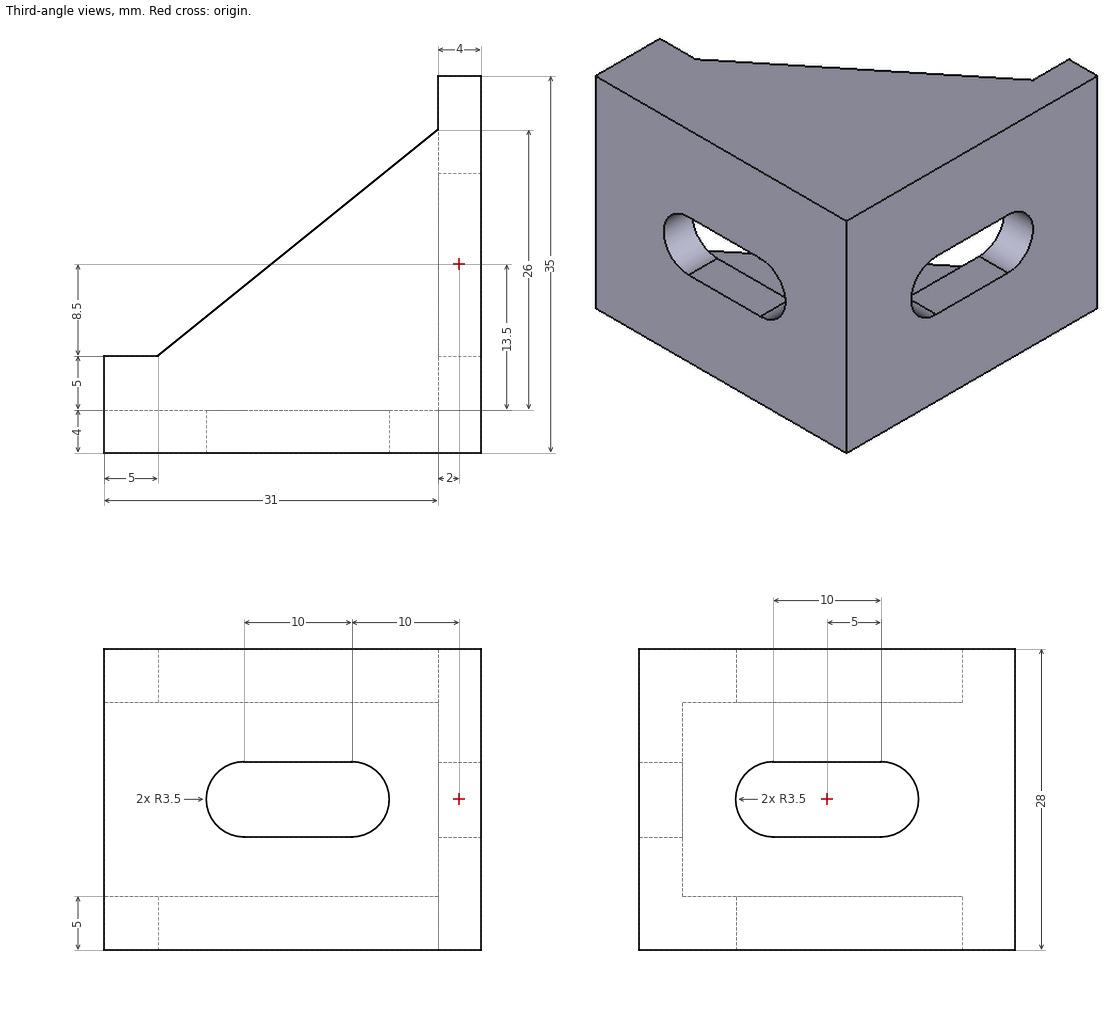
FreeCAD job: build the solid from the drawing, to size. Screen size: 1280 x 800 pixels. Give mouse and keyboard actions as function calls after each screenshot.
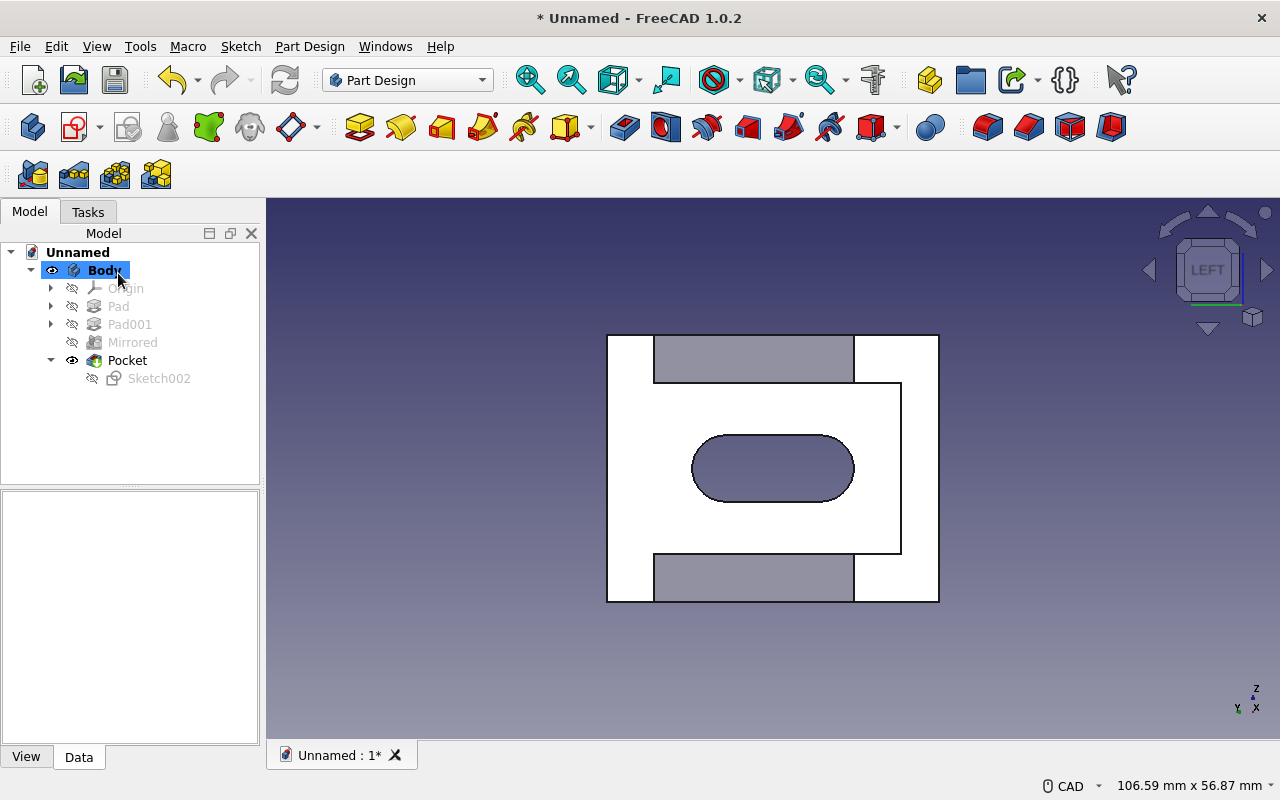
key(4)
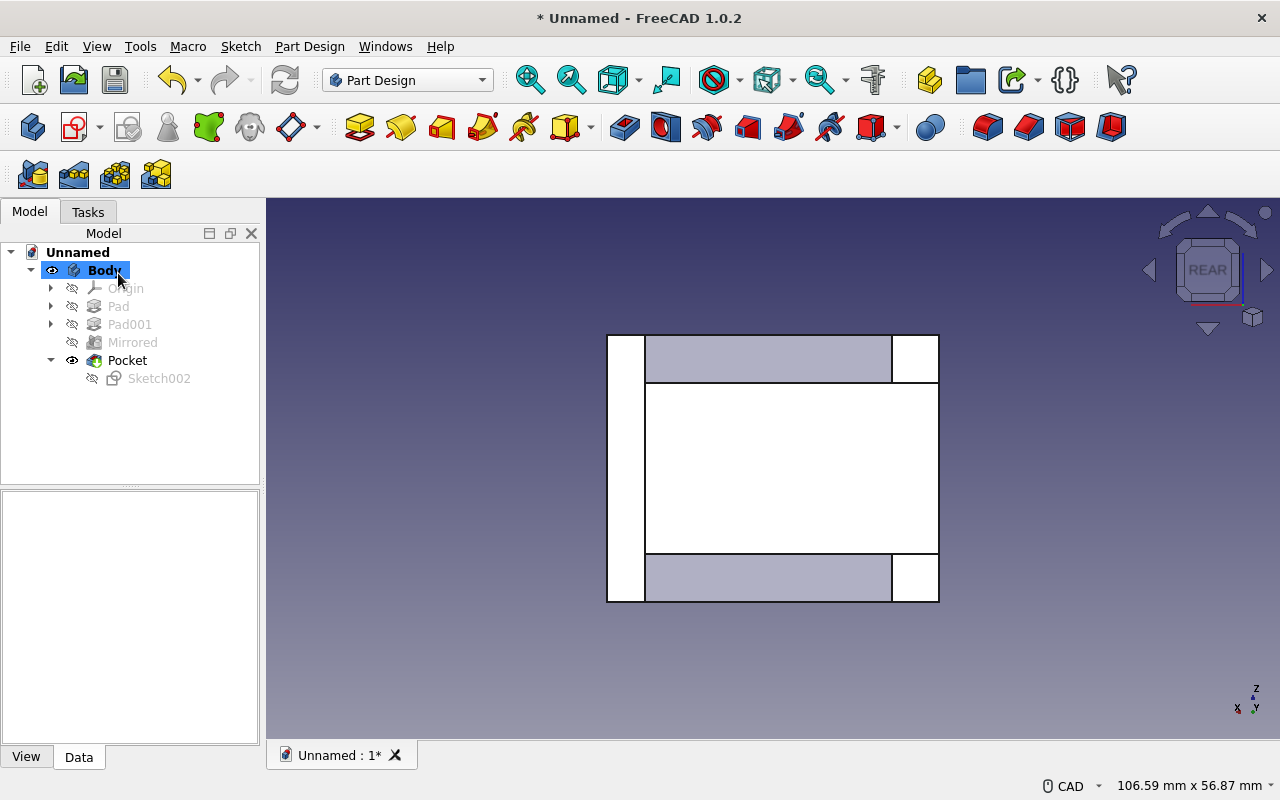
click(750, 468)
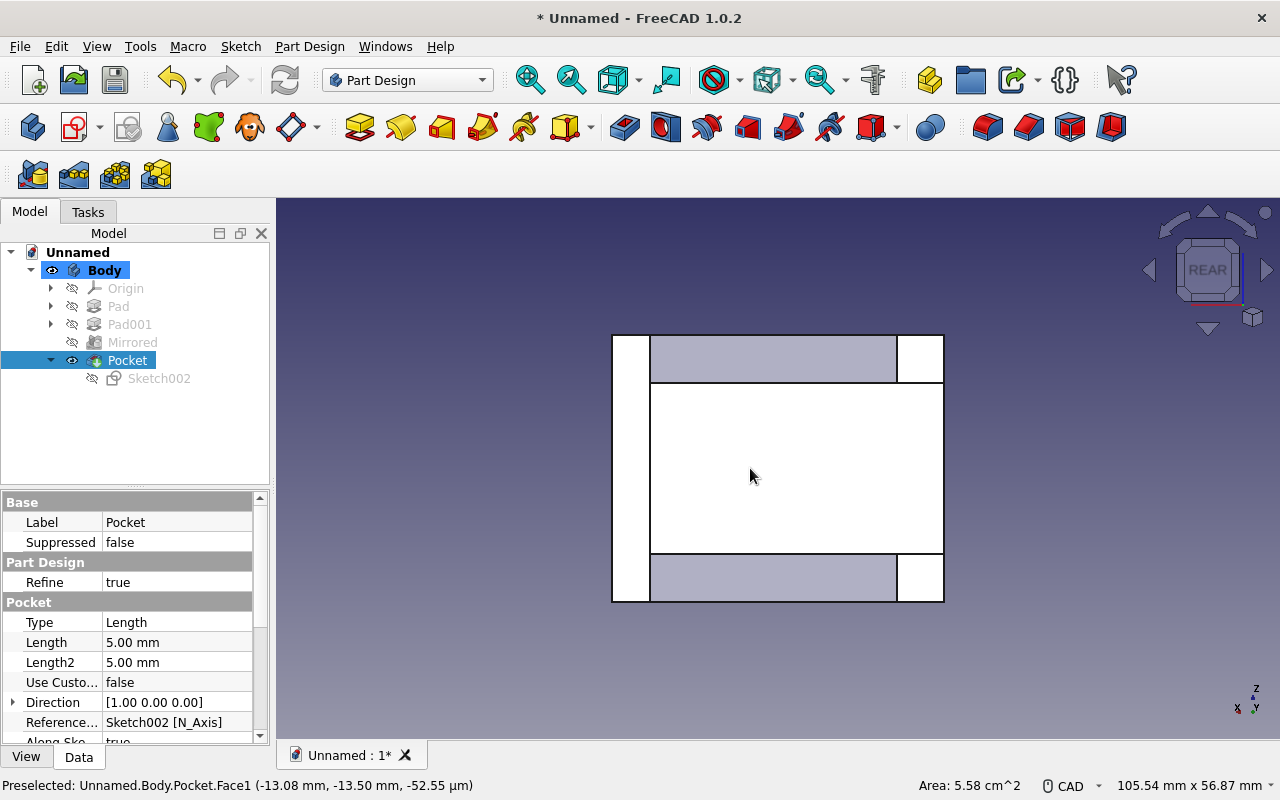
click(74, 128)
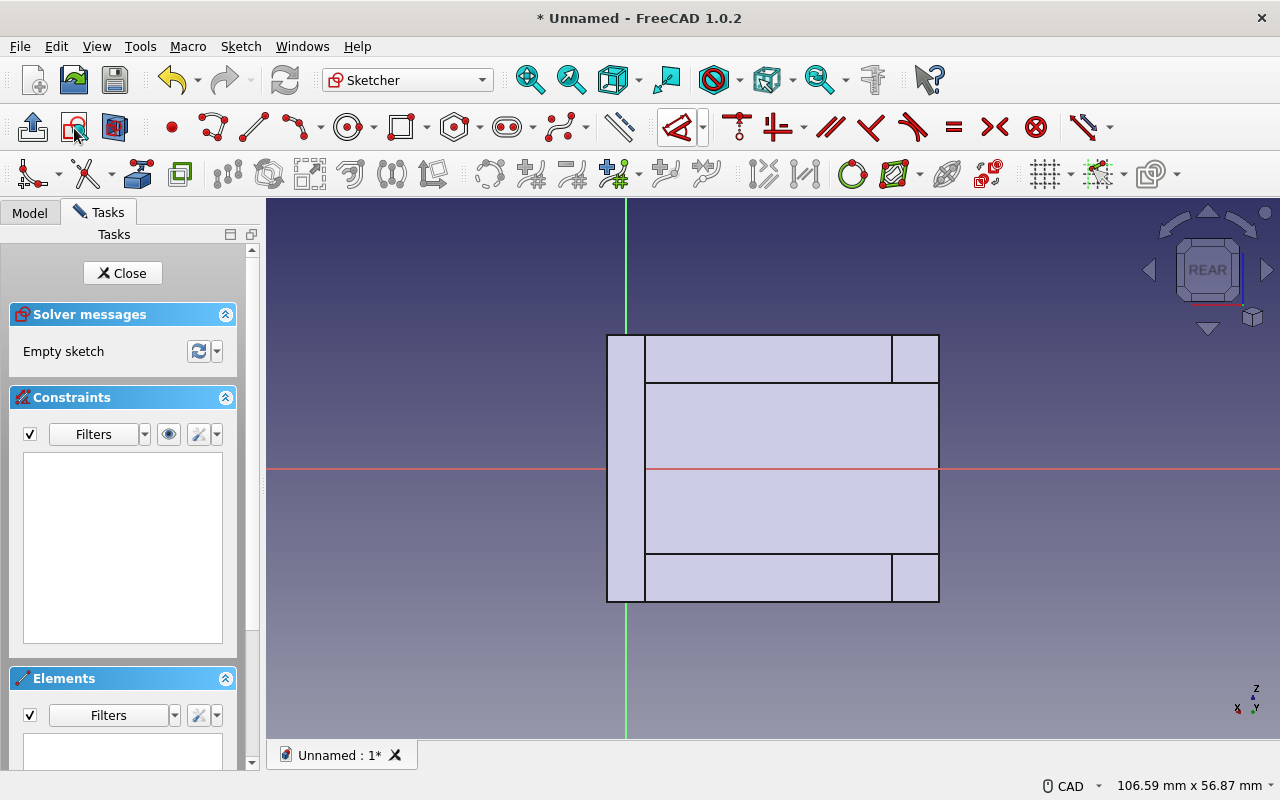
click(115, 128)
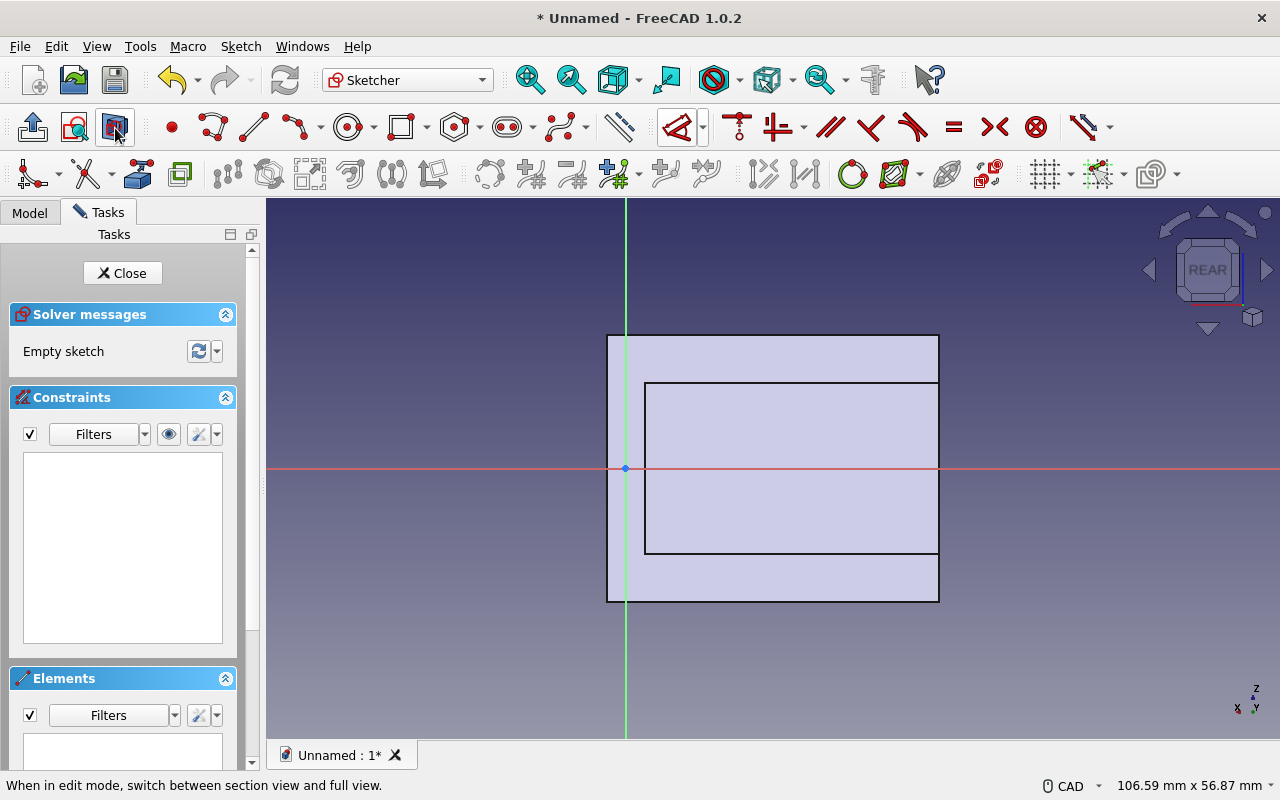
scroll(756, 469, up, 5)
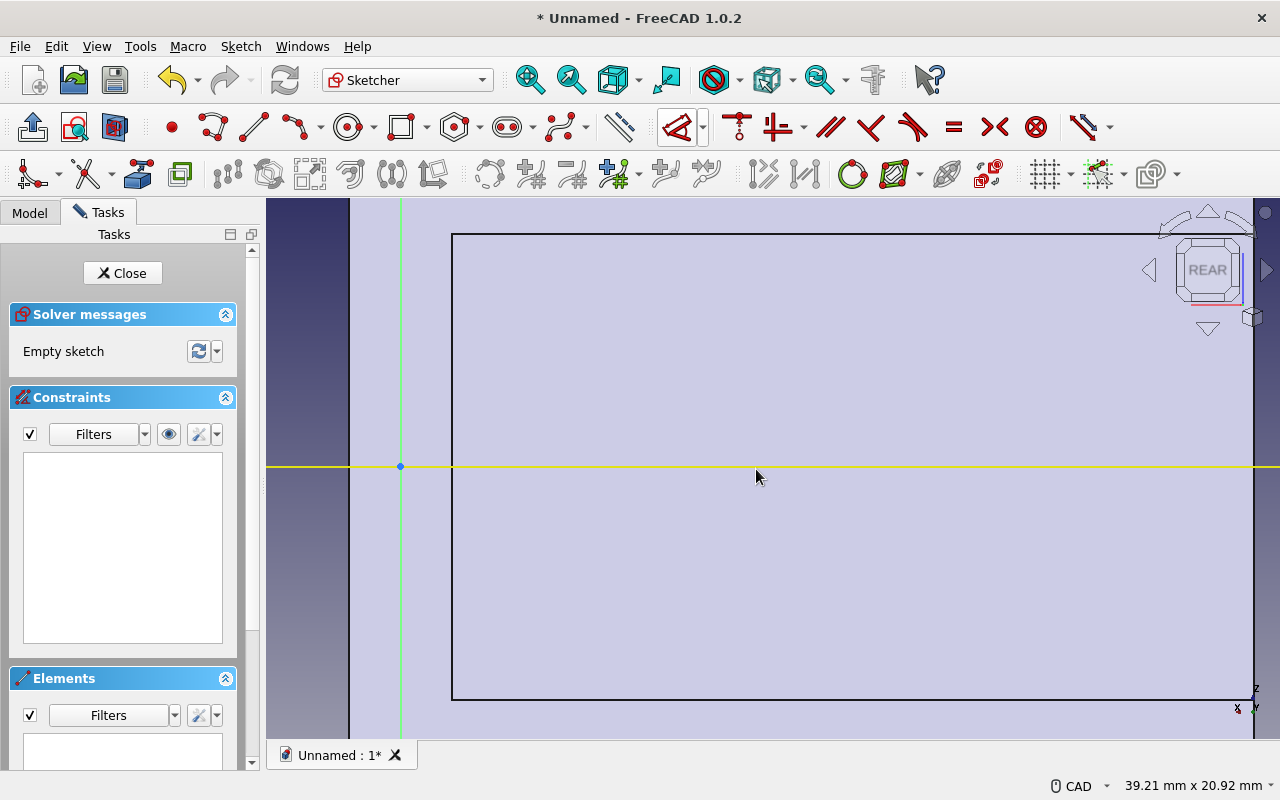
click(506, 128)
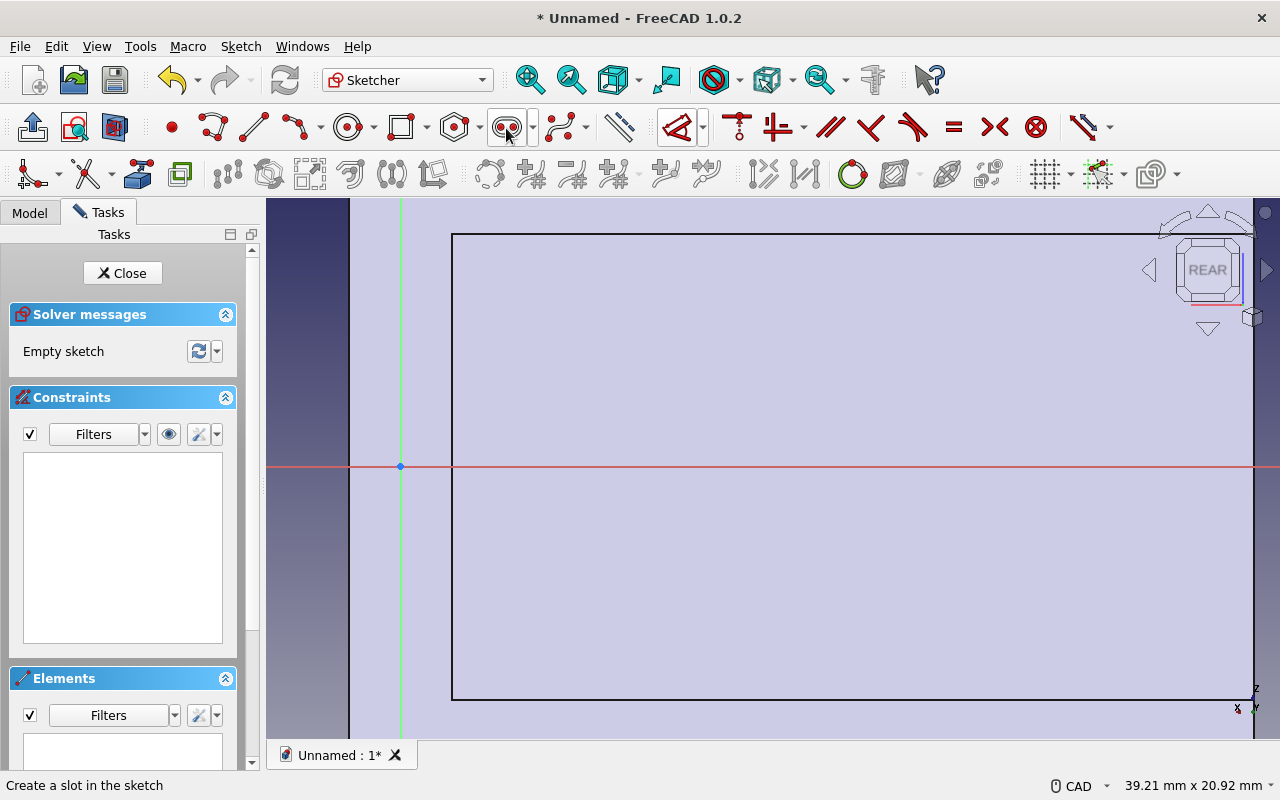
click(659, 467)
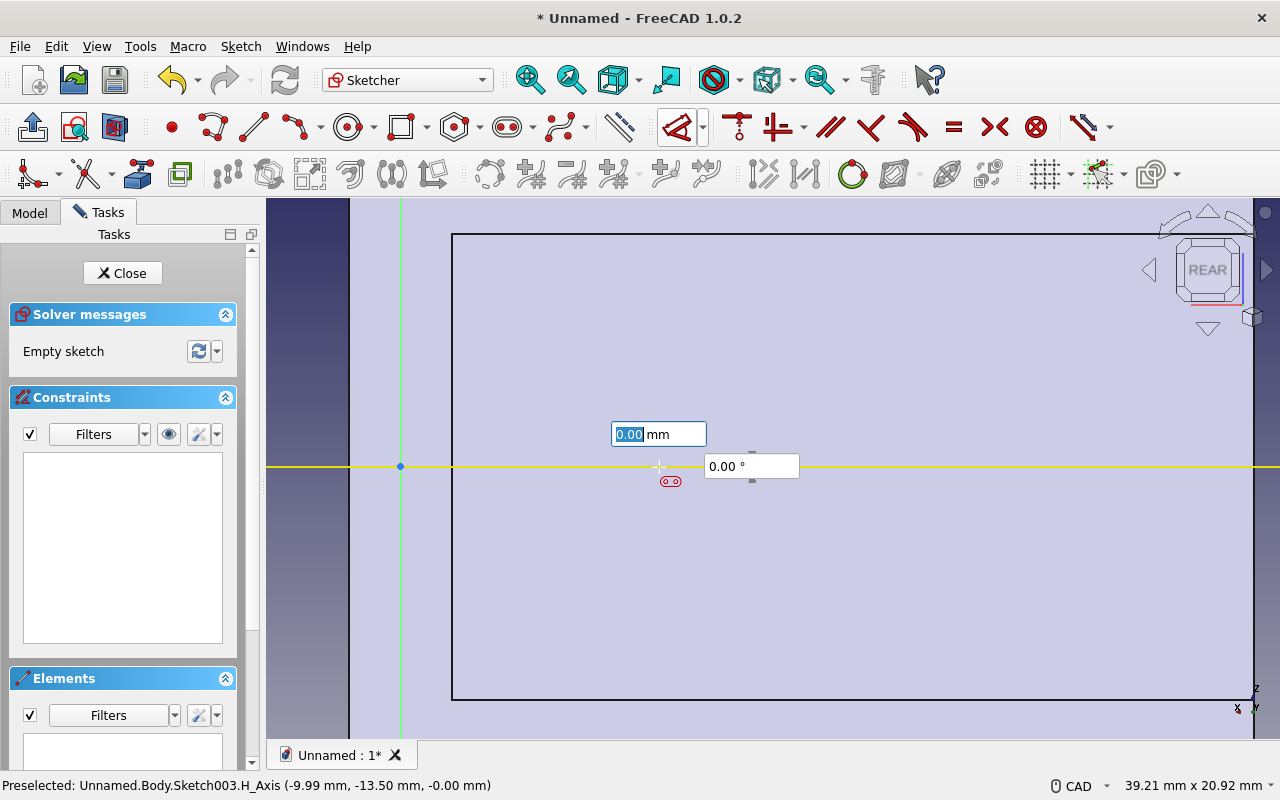
click(918, 458)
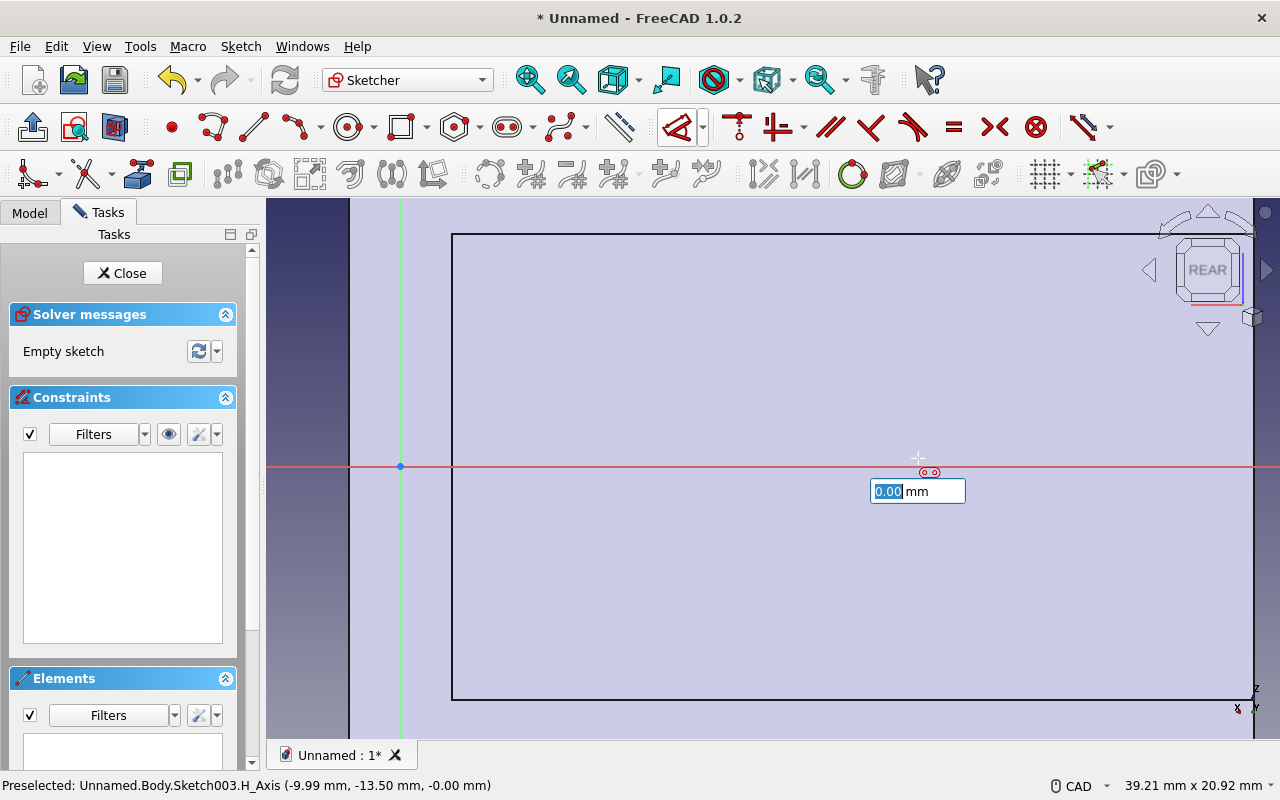
click(788, 557)
key(Escape)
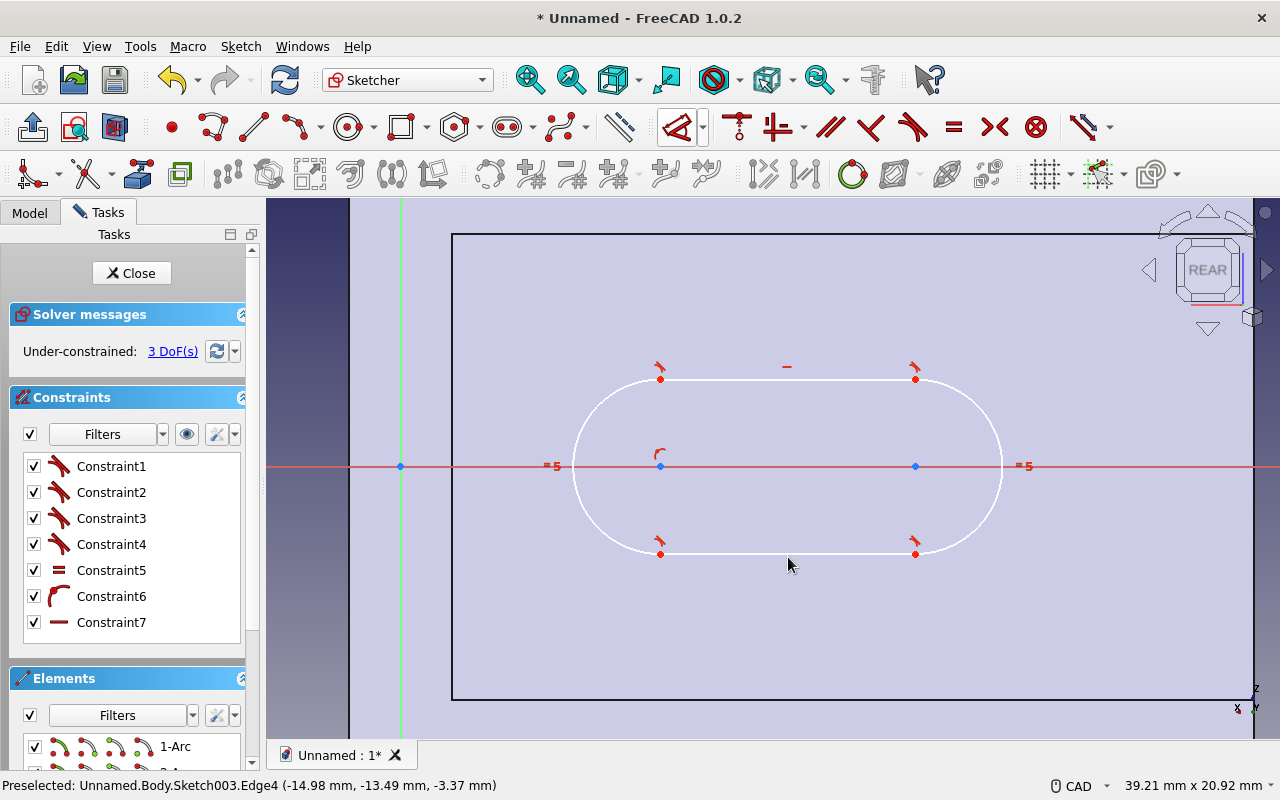
click(590, 416)